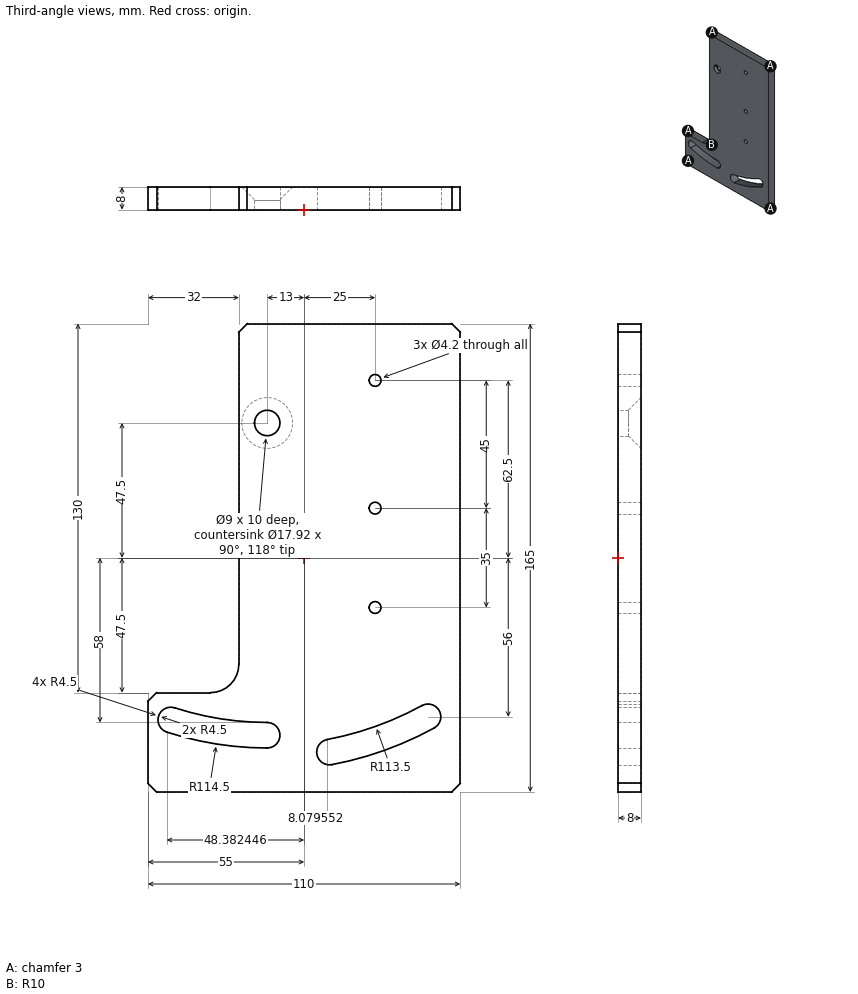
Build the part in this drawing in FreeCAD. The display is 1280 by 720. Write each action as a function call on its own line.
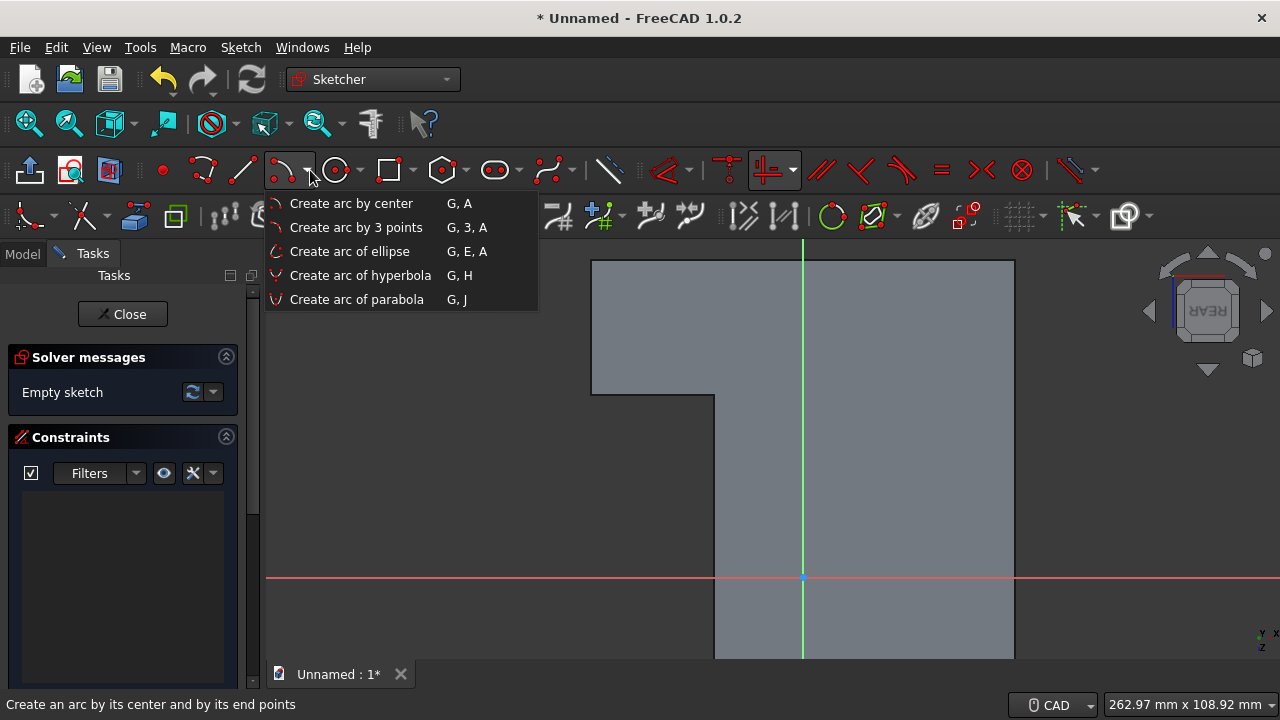
click(402, 227)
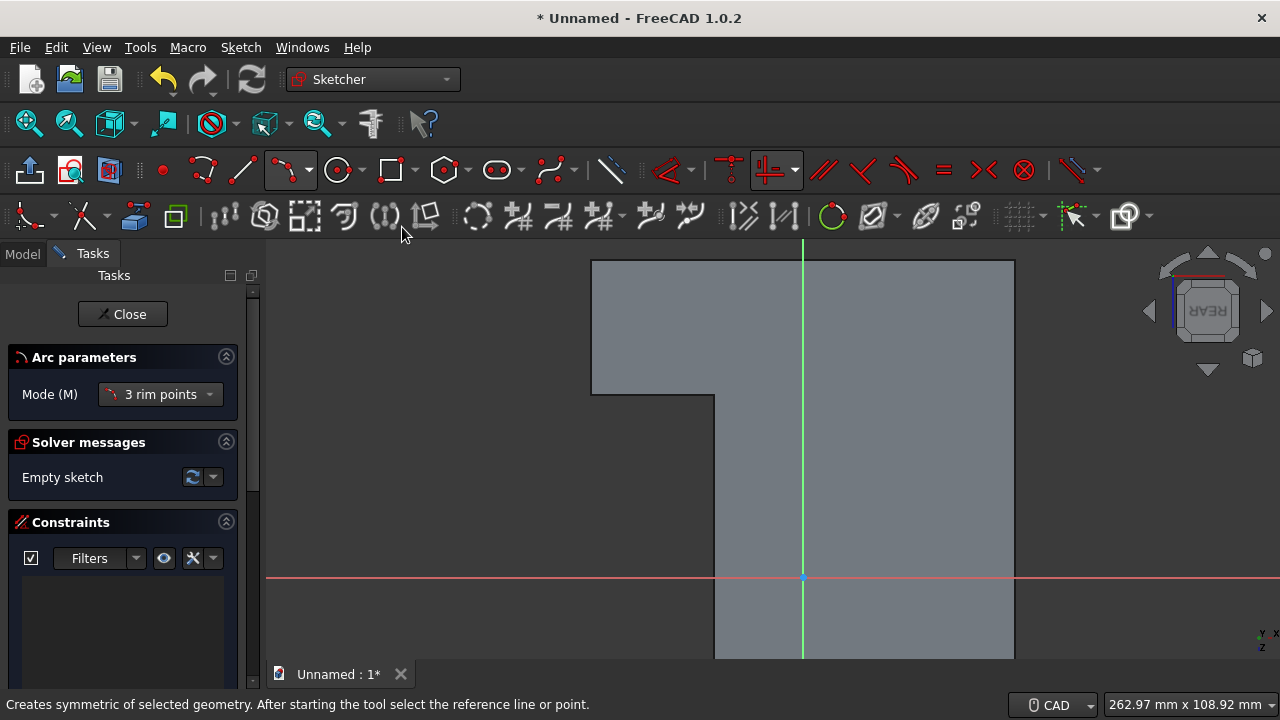
click(753, 354)
click(753, 320)
click(770, 337)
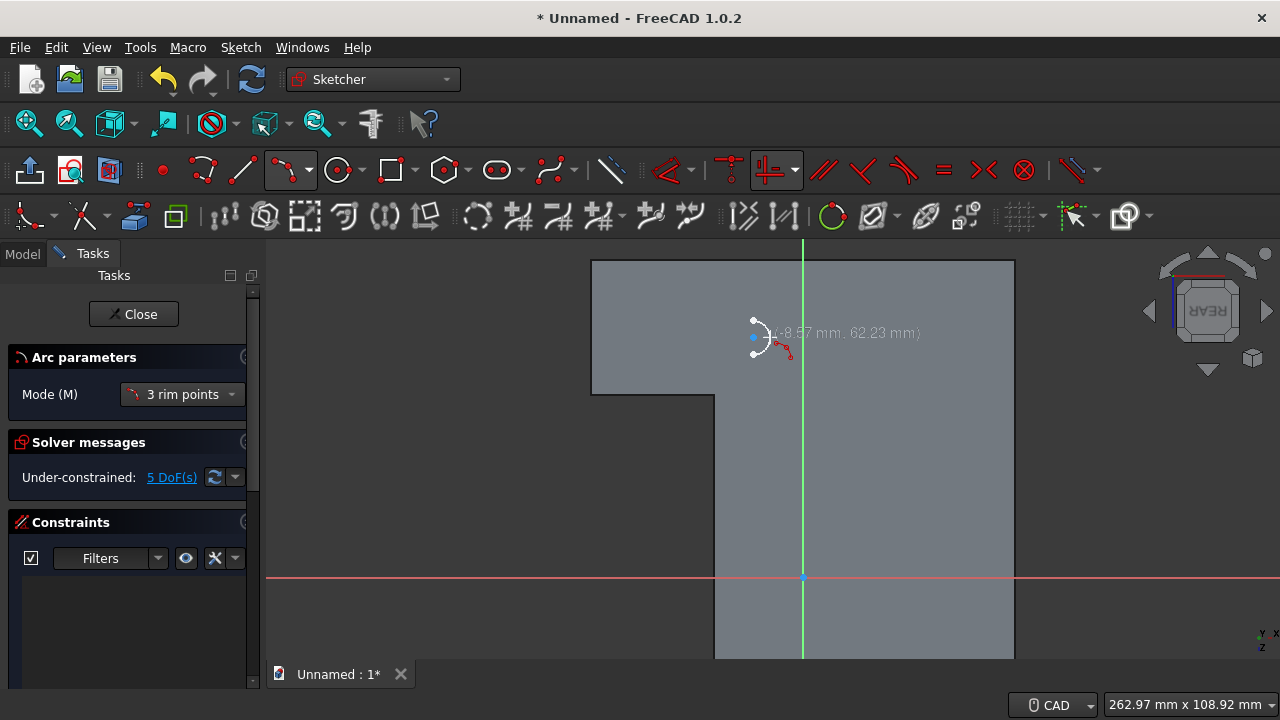
click(753, 321)
click(616, 341)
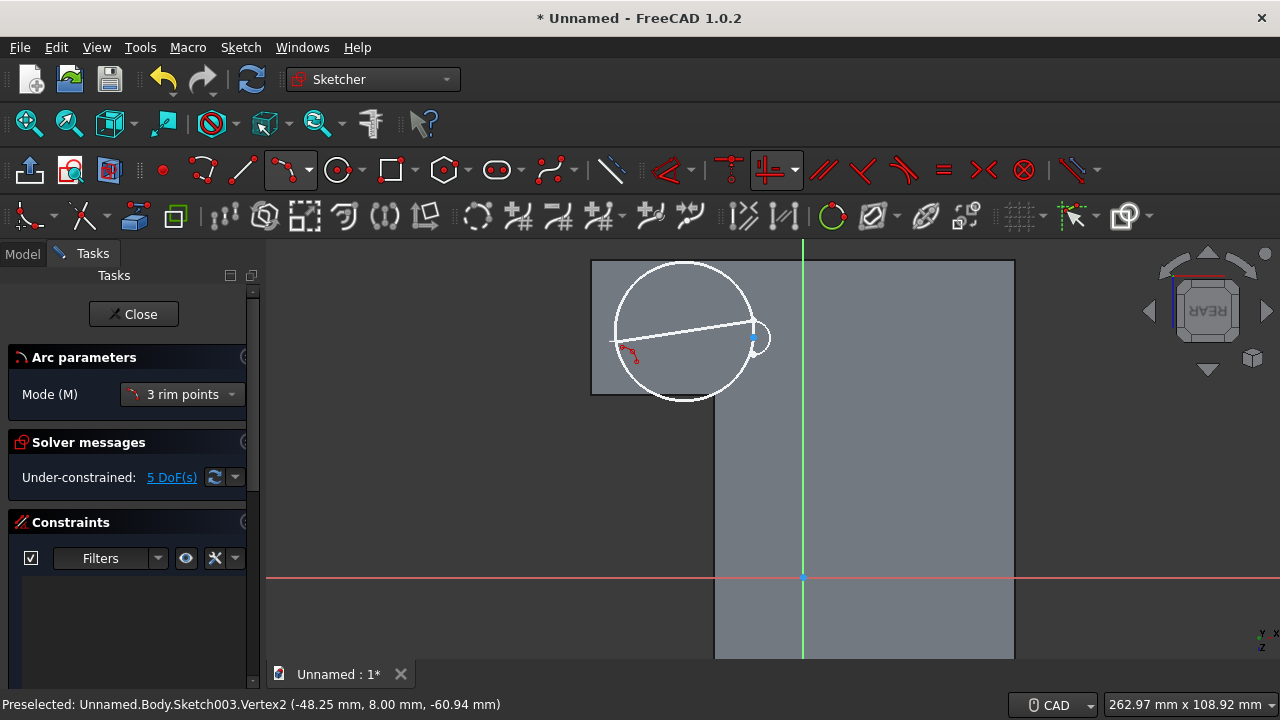
scroll(684, 325, up, 6)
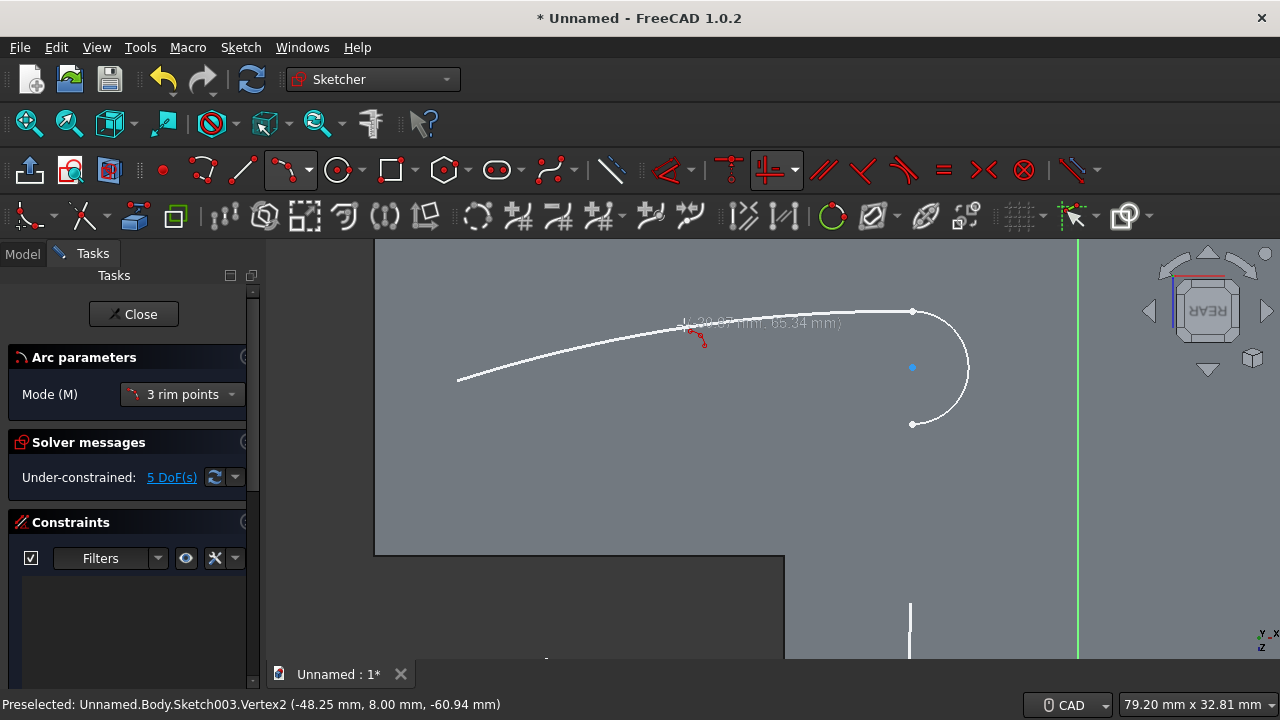
click(683, 325)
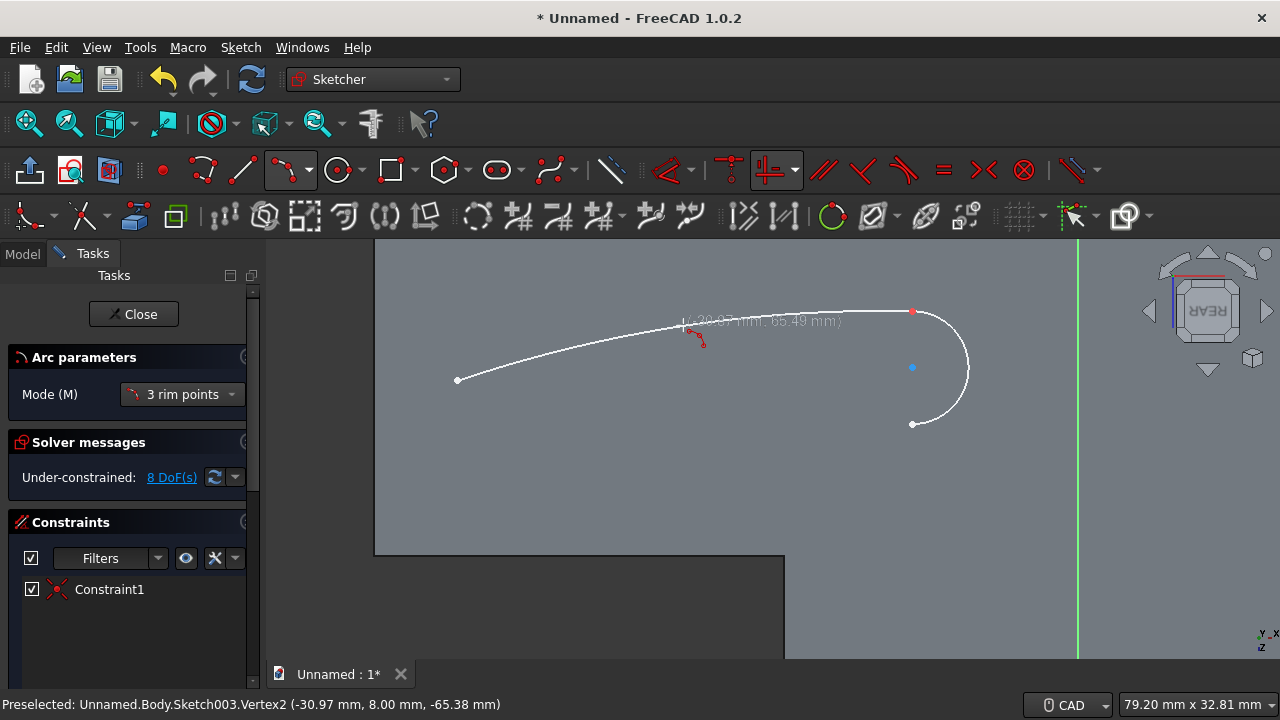
click(457, 381)
click(494, 488)
click(422, 451)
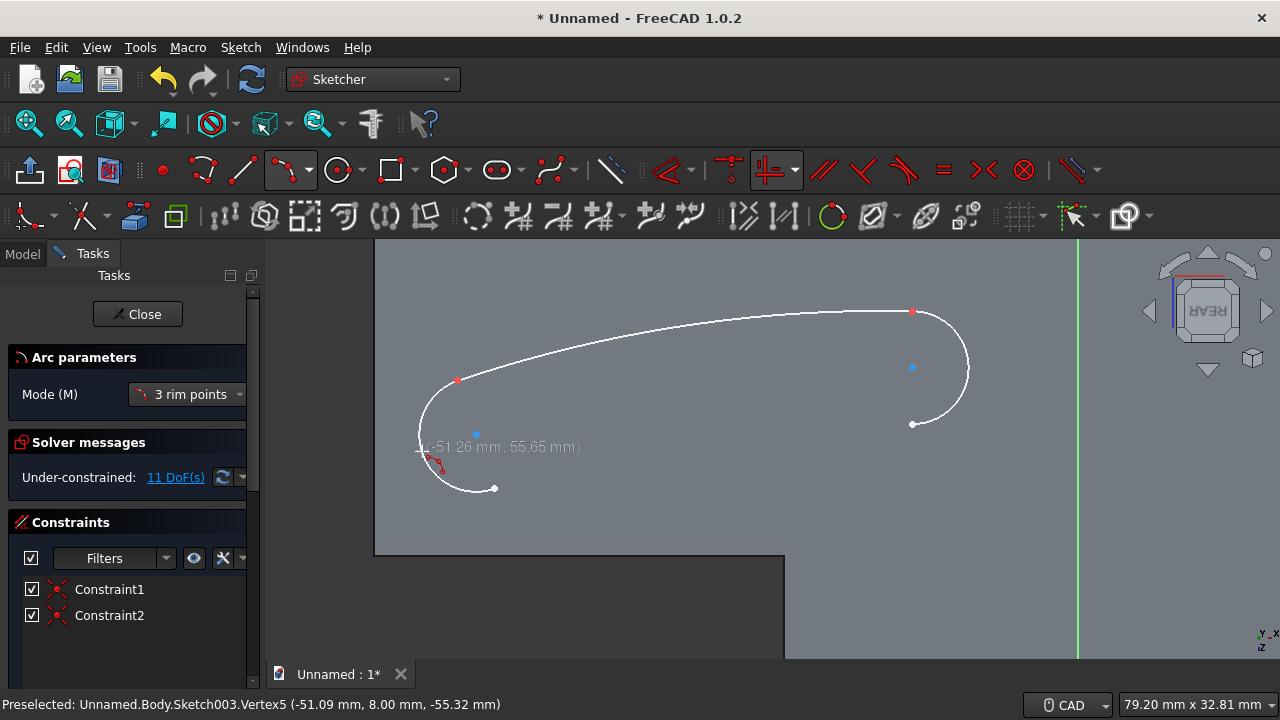
click(494, 489)
click(912, 424)
click(701, 438)
key(Escape)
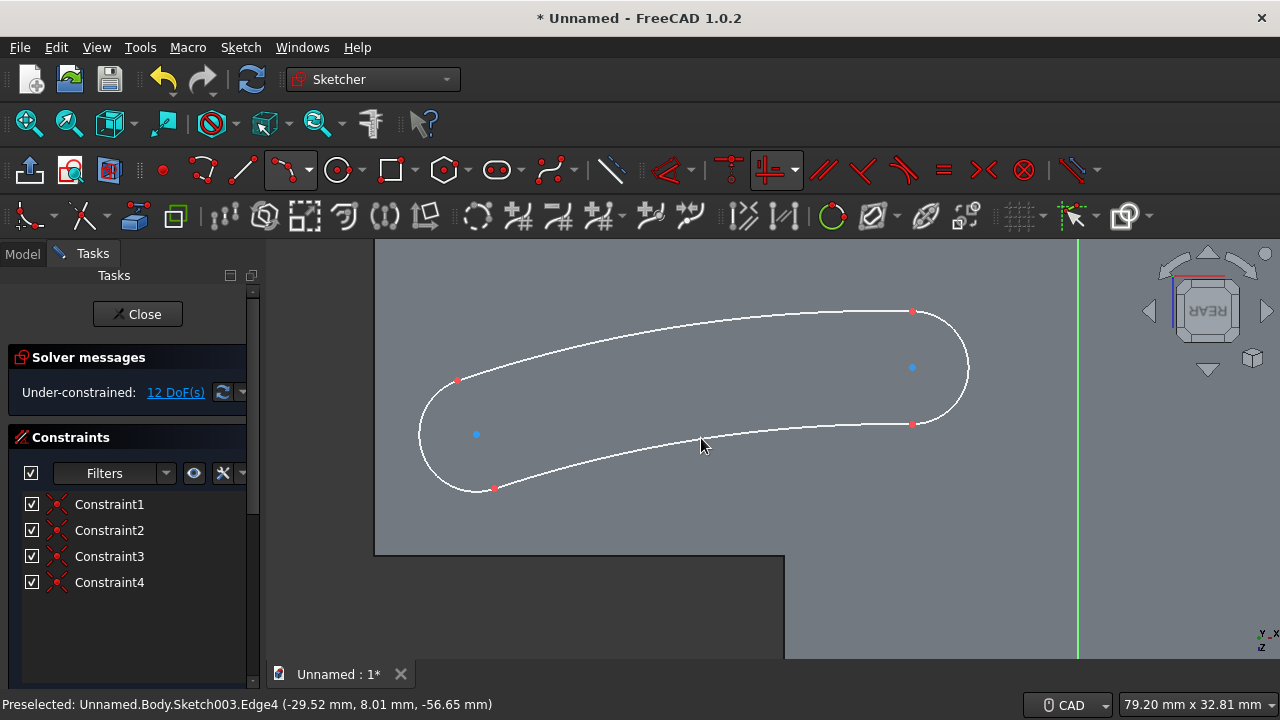
click(958, 401)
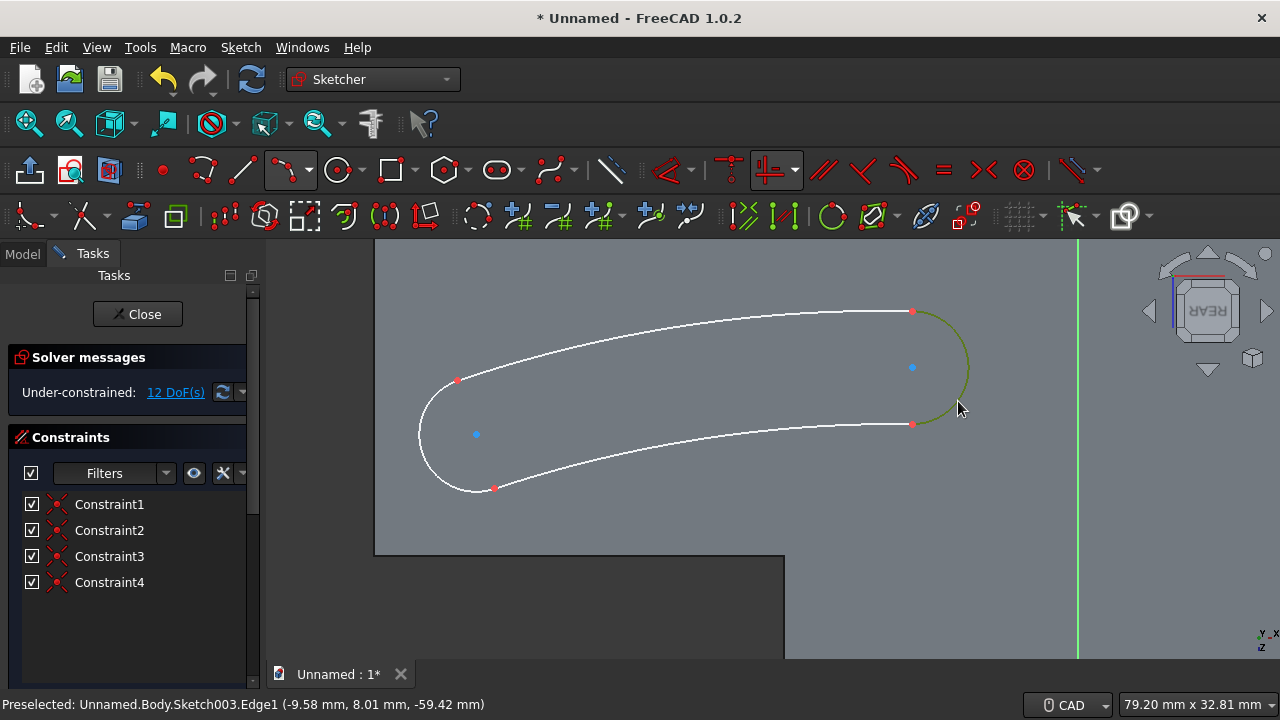
click(774, 315)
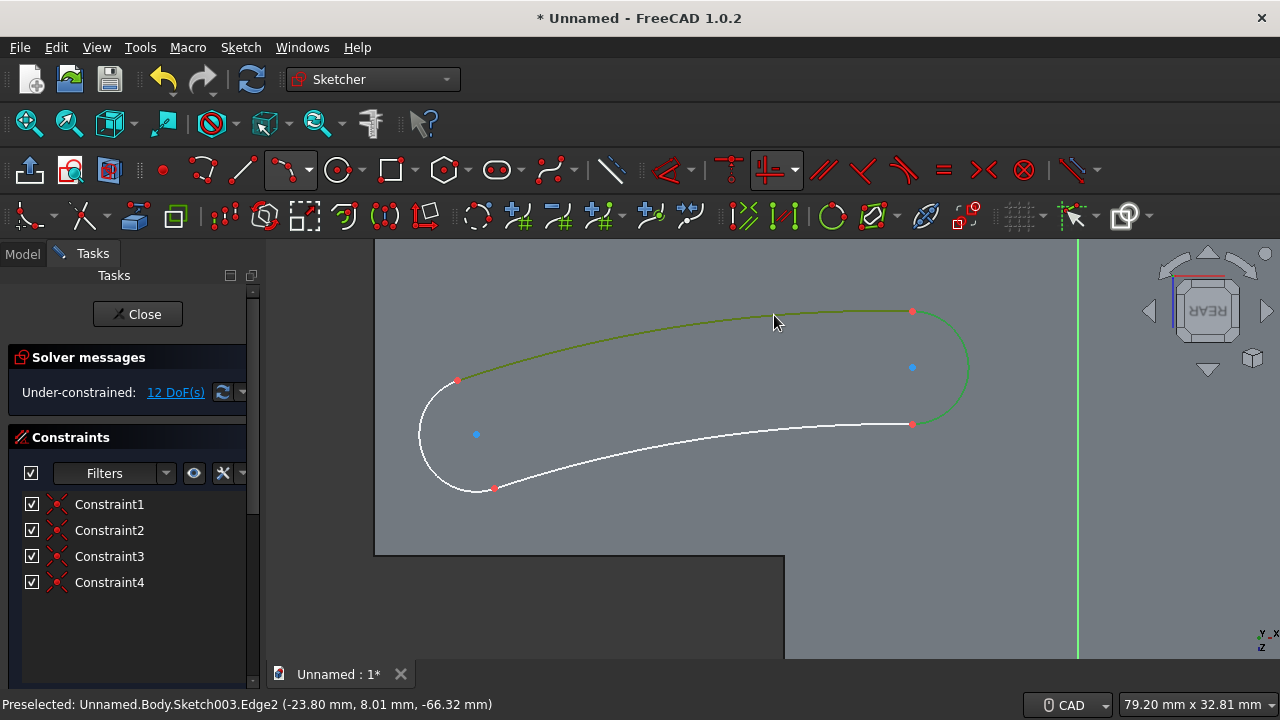
click(904, 170)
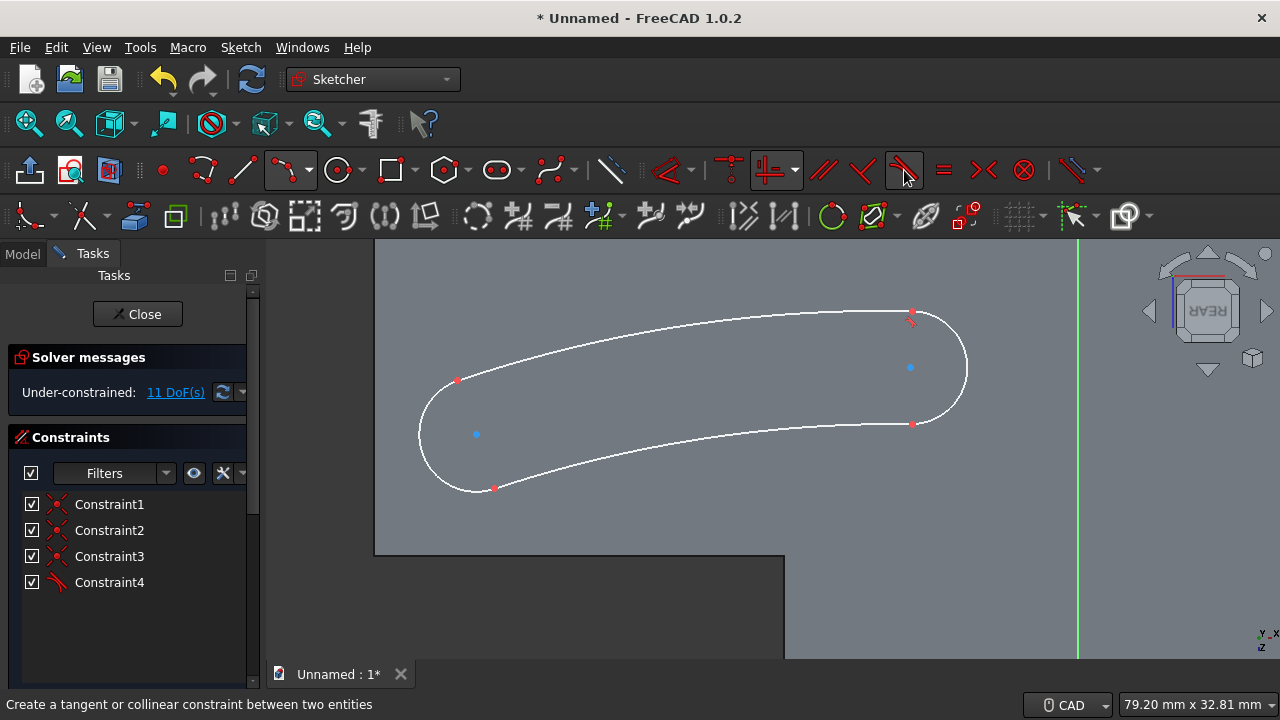
click(957, 400)